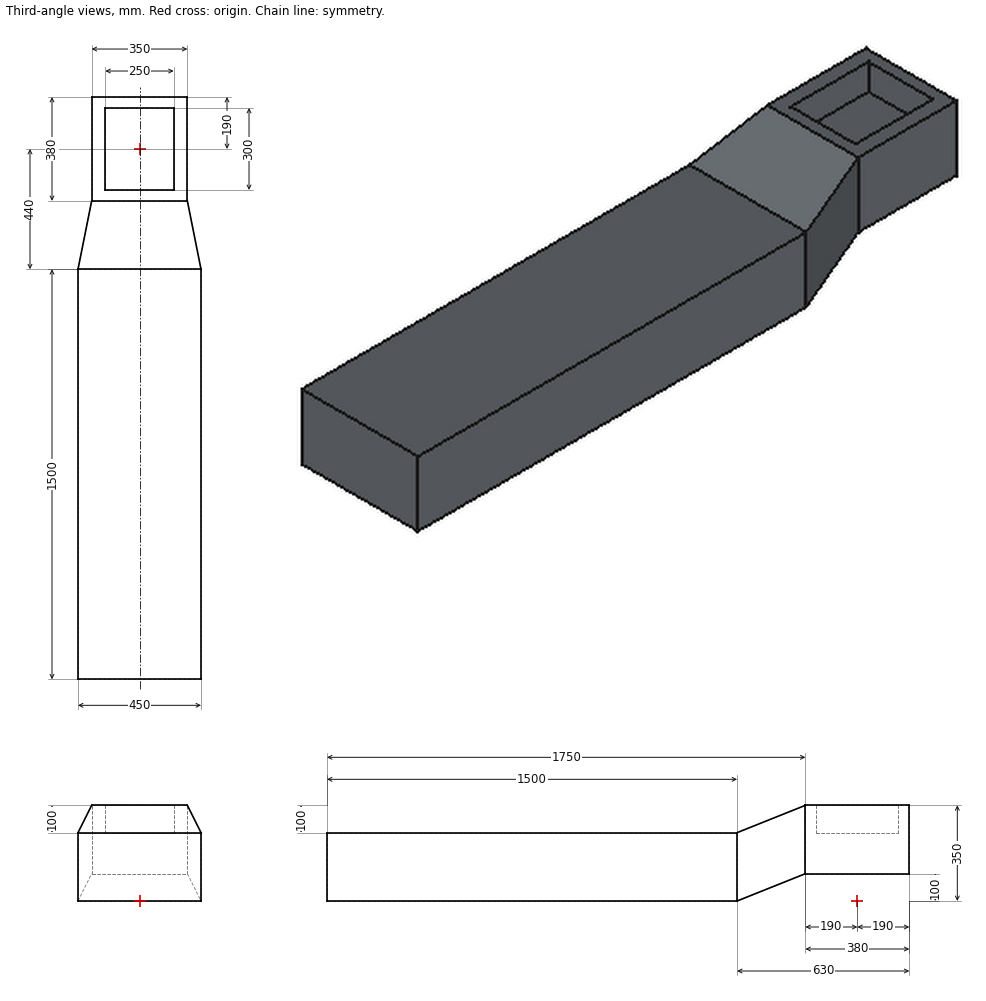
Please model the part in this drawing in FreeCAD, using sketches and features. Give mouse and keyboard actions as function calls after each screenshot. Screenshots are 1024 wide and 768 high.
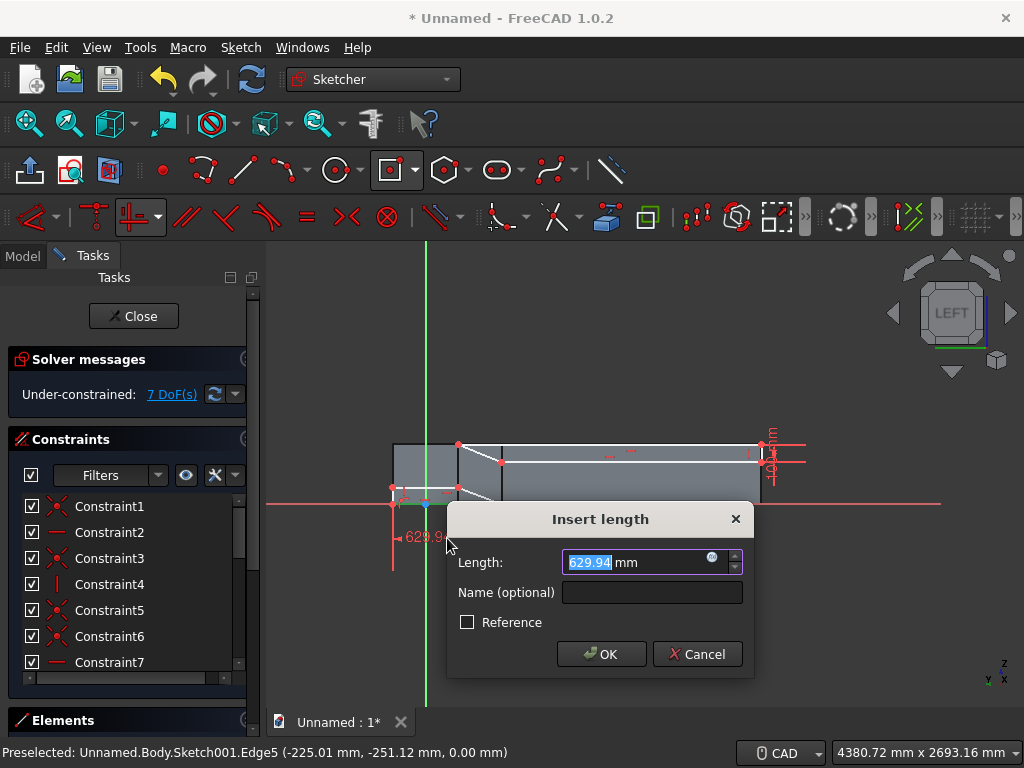
text(630)
key(Return)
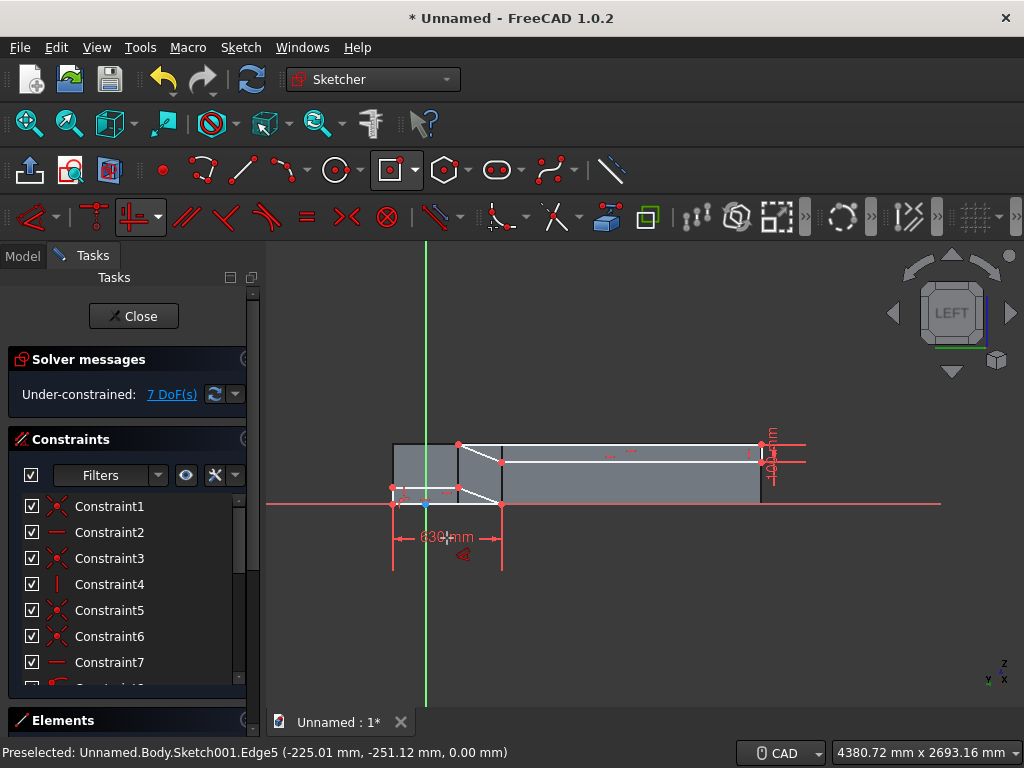
click(439, 488)
click(410, 454)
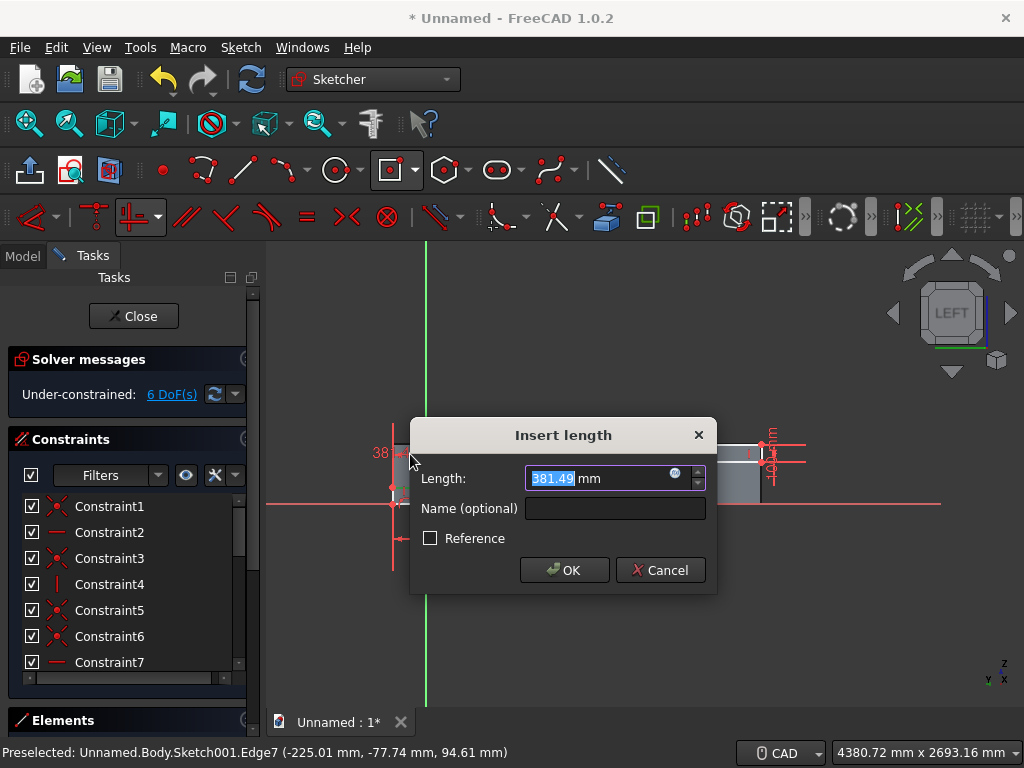
text(380)
key(Return)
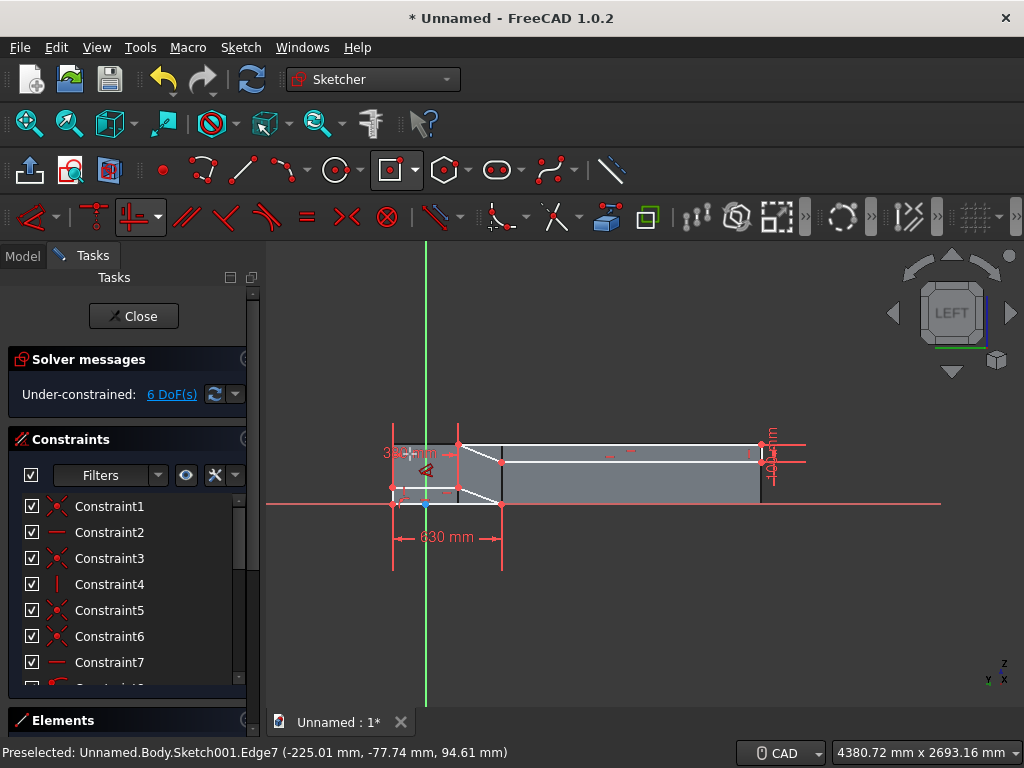
scroll(393, 496, up, 5)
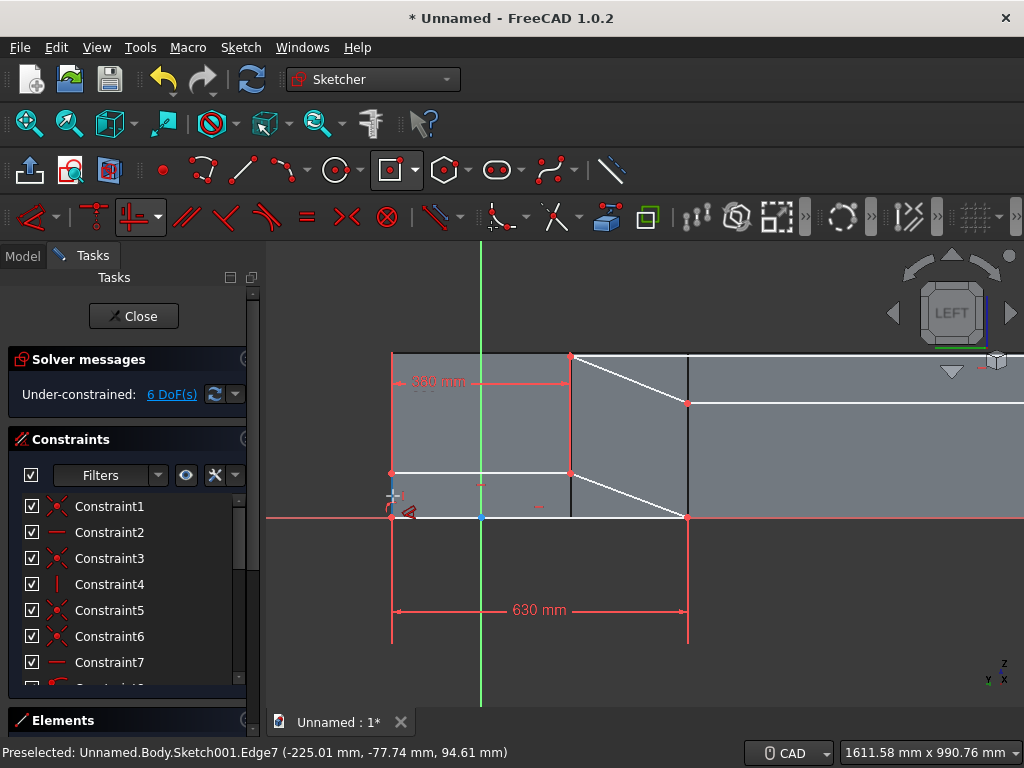
click(392, 496)
click(358, 496)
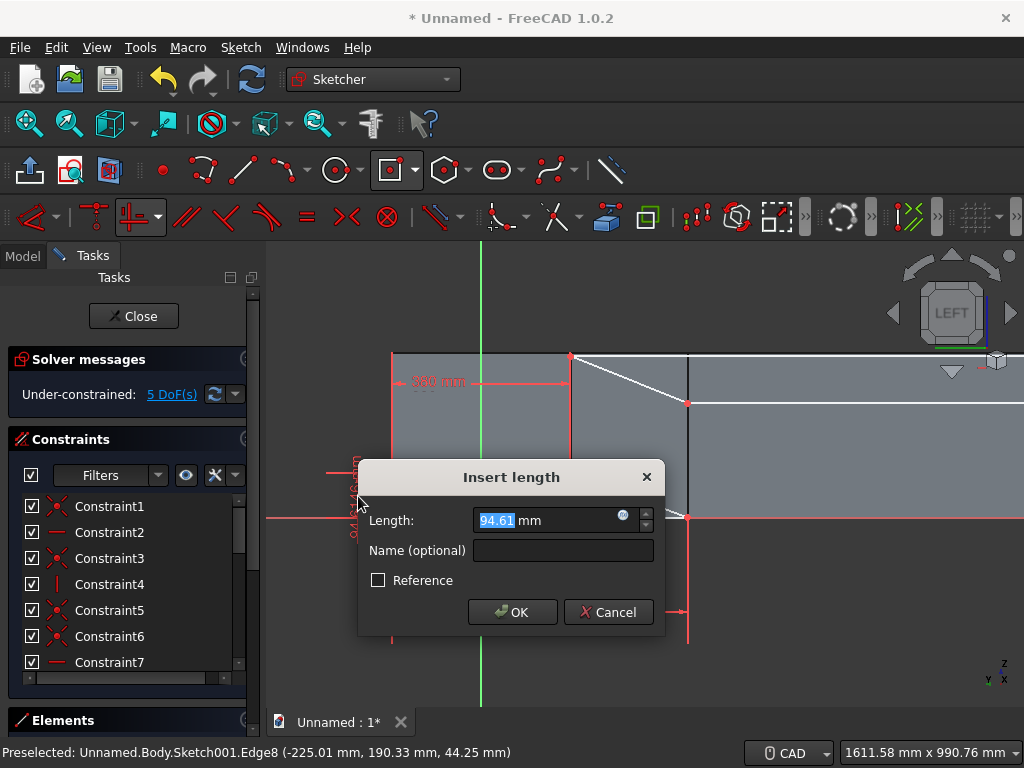
text(100)
key(Return)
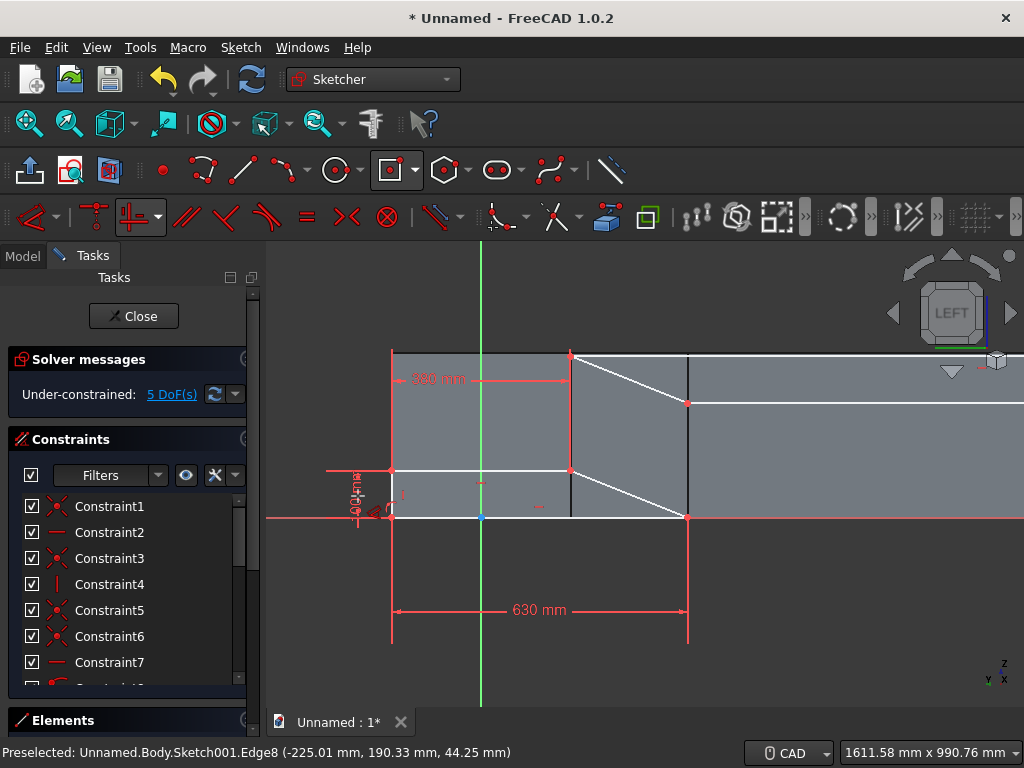
click(829, 403)
click(773, 369)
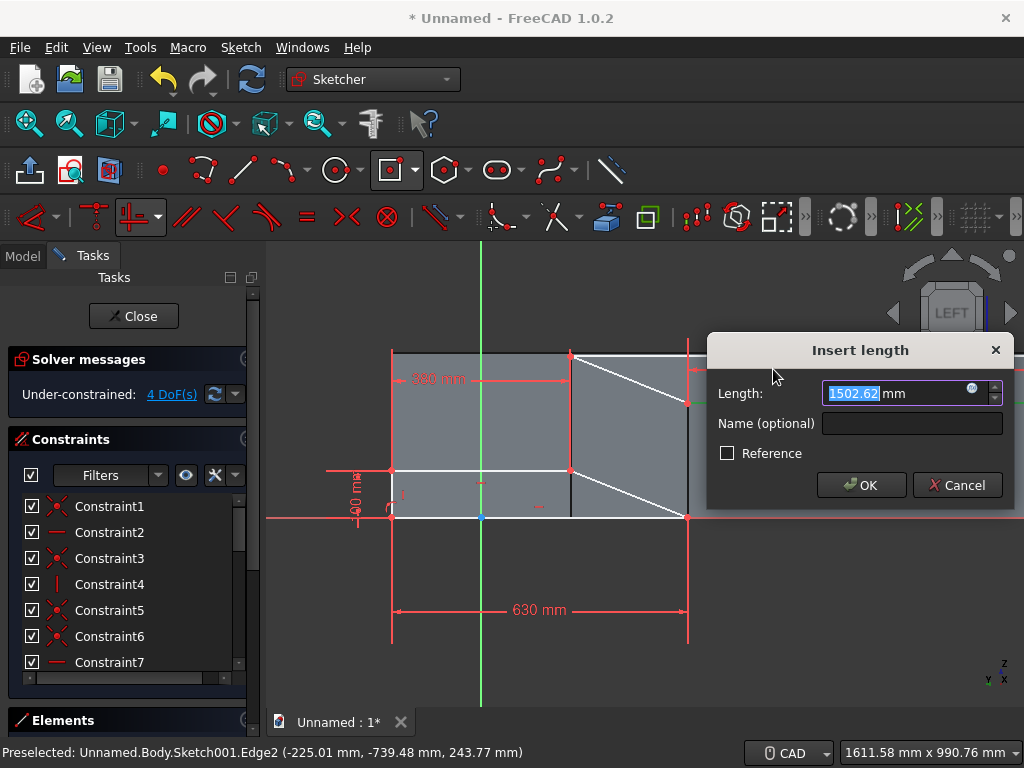
text(1500)
key(Return)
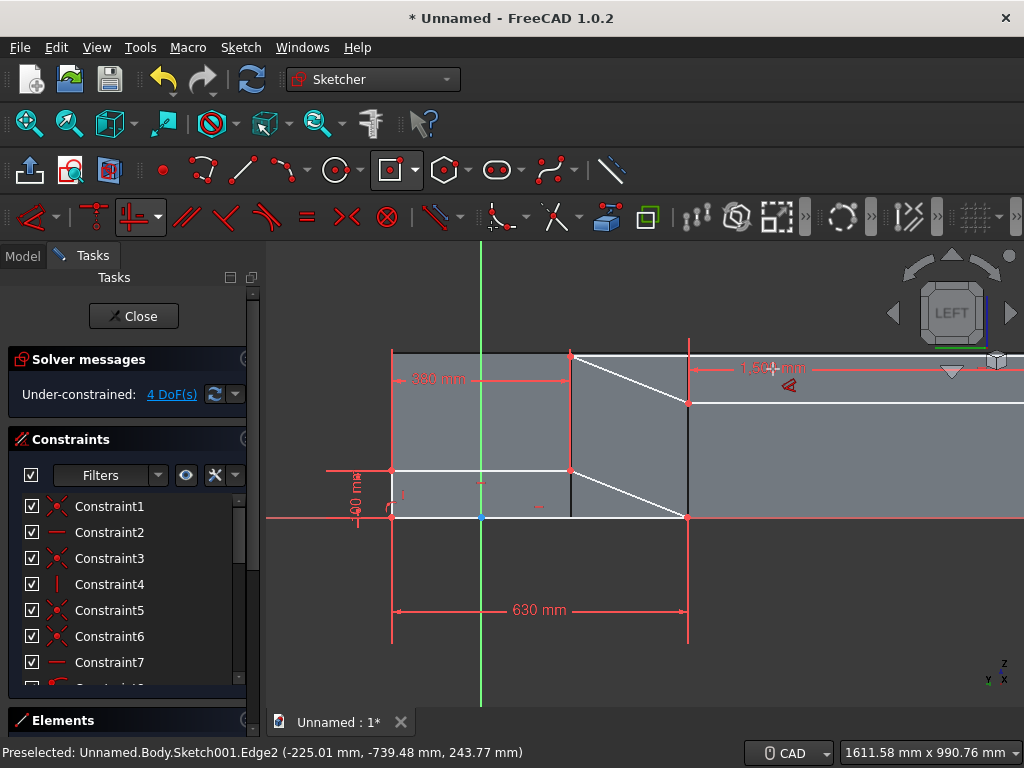
click(818, 356)
click(715, 322)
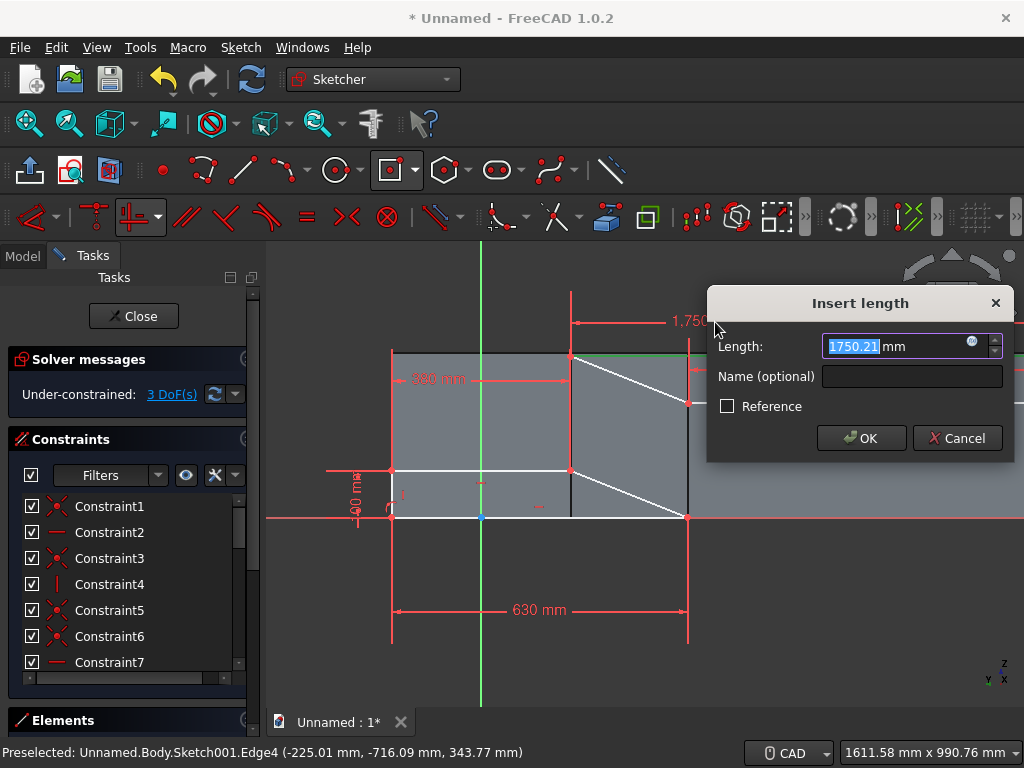
text(1750)
key(Return)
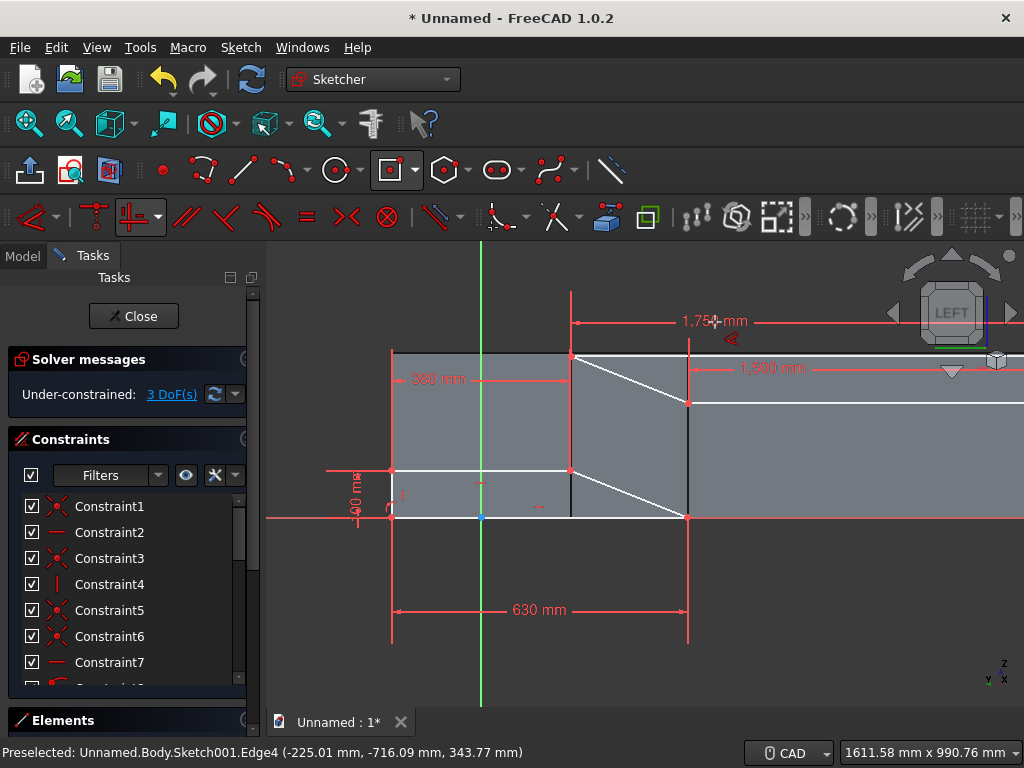
click(571, 356)
click(526, 552)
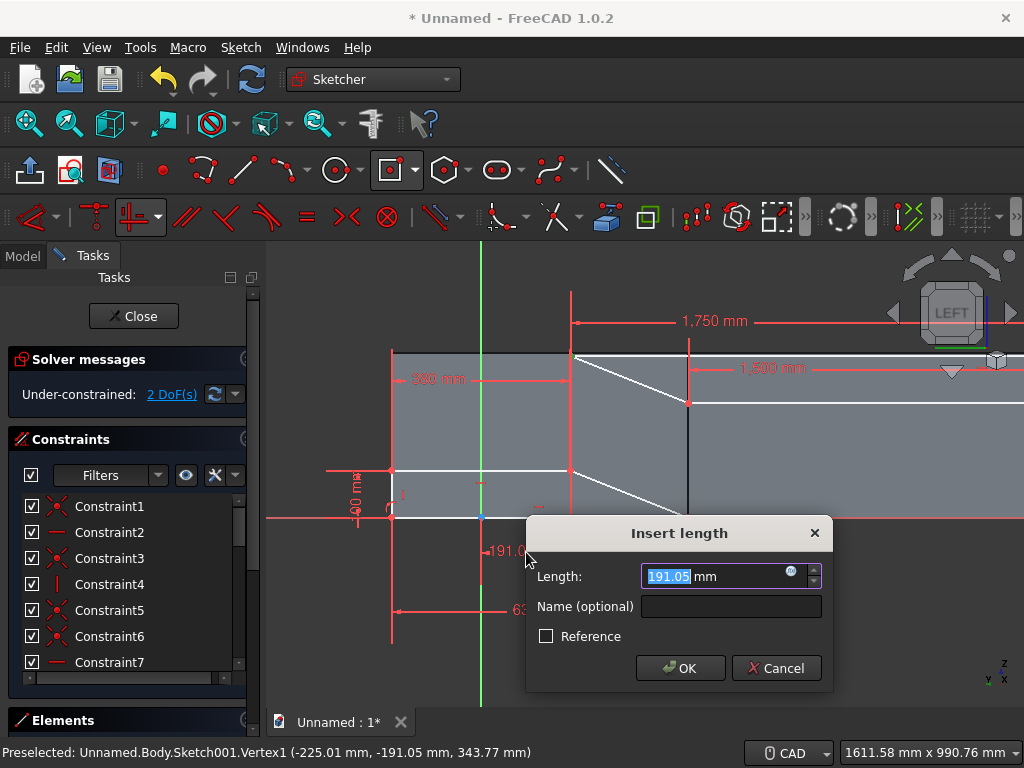
text(190)
key(Return)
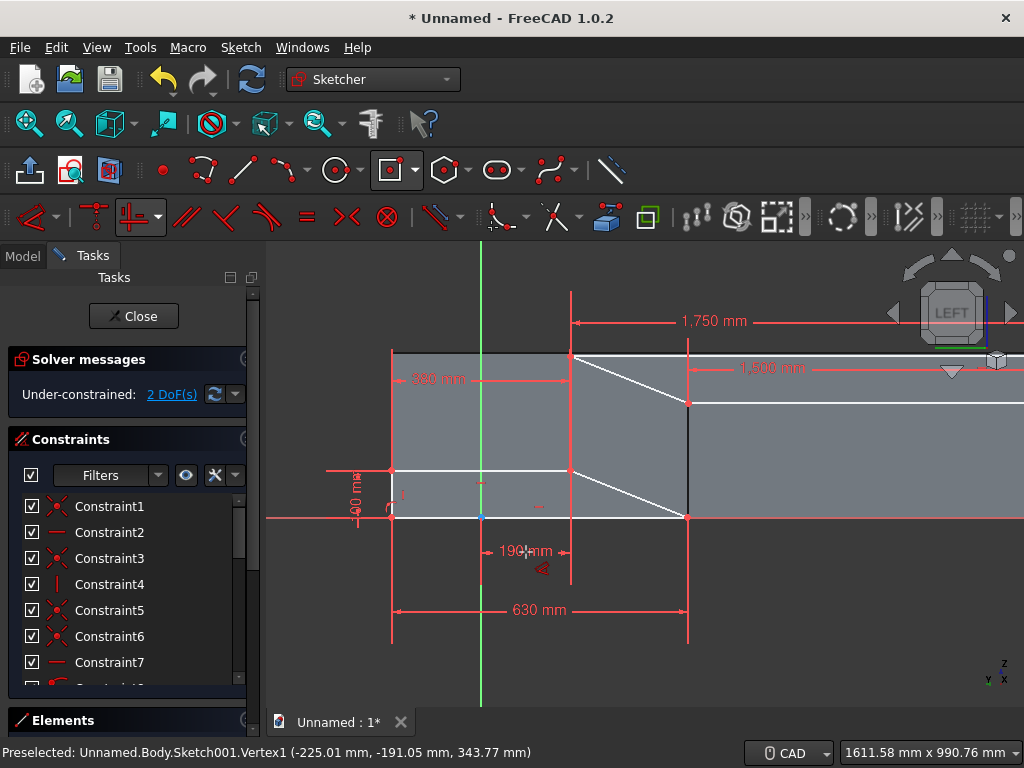
click(571, 356)
click(447, 437)